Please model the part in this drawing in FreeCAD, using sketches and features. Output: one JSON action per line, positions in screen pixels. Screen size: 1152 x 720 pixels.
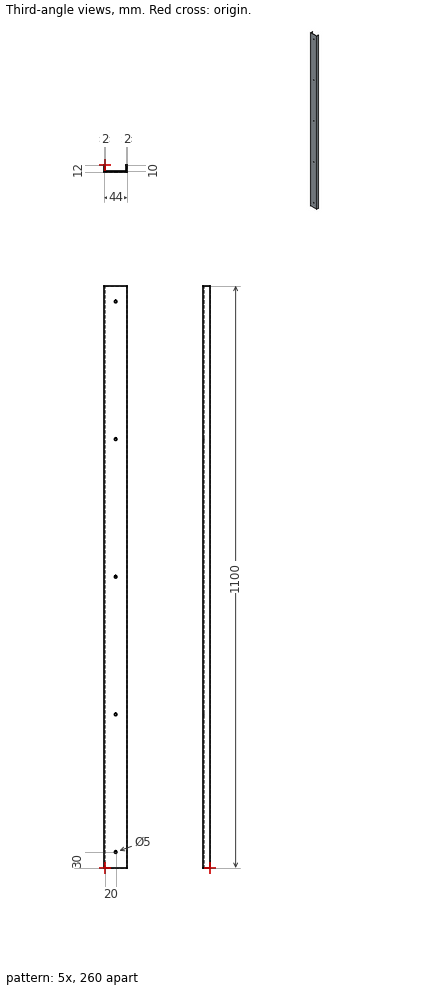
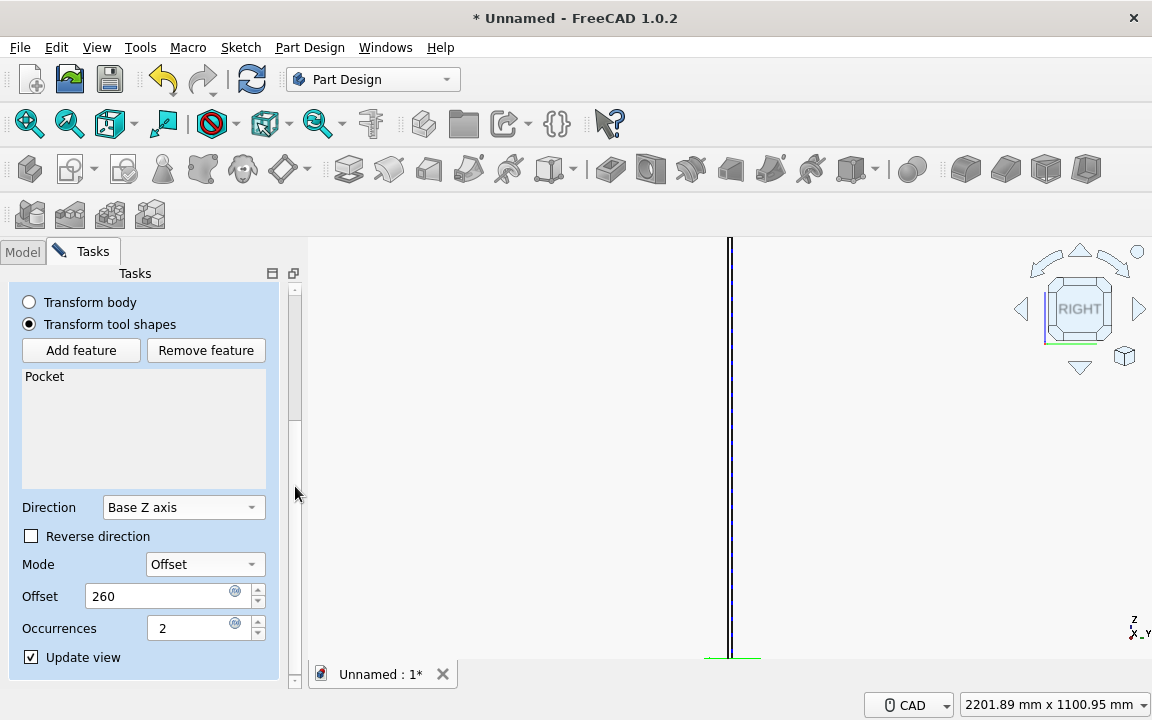
{"action": "triple_click", "coordinate": [198, 628]}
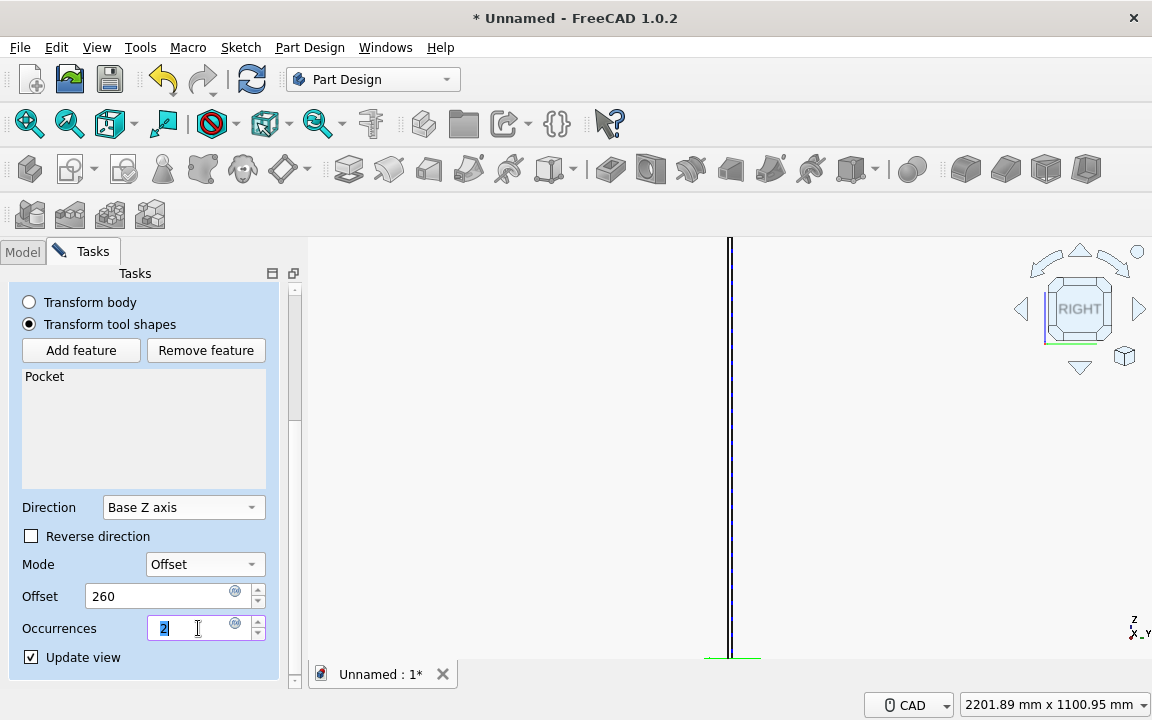
{"action": "type", "text": "5"}
{"action": "key", "text": "Tab"}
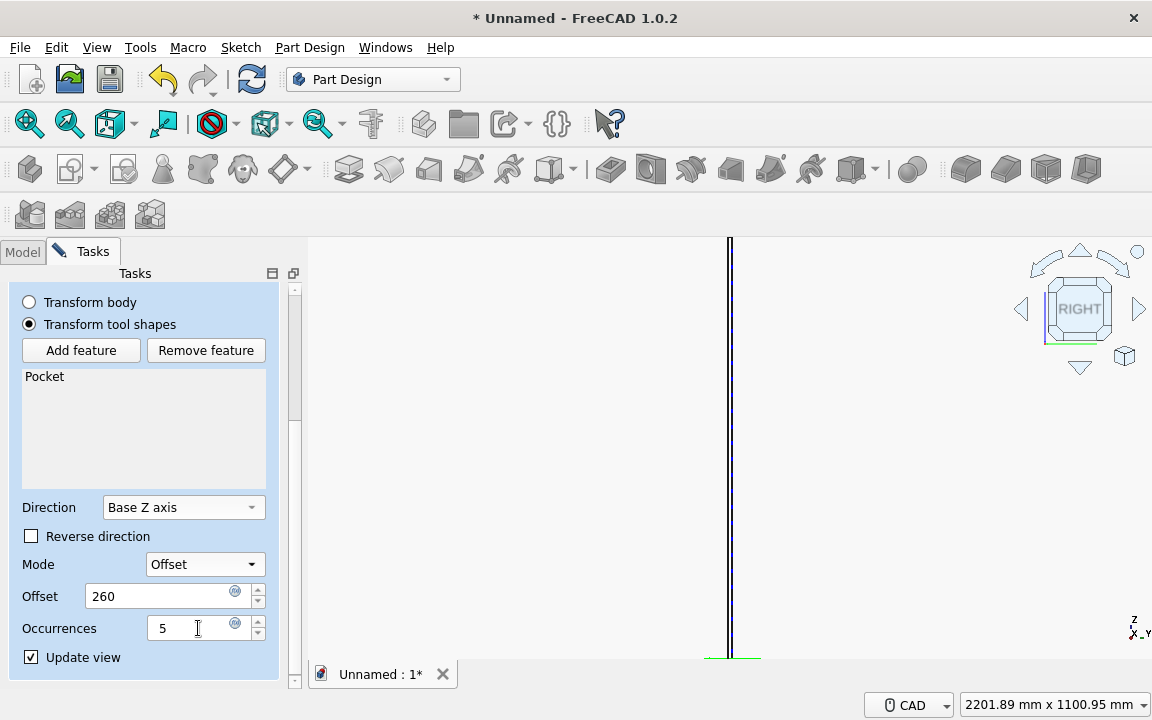
{"action": "scroll", "coordinate": [295, 486], "scroll_direction": "up", "scroll_amount": 5}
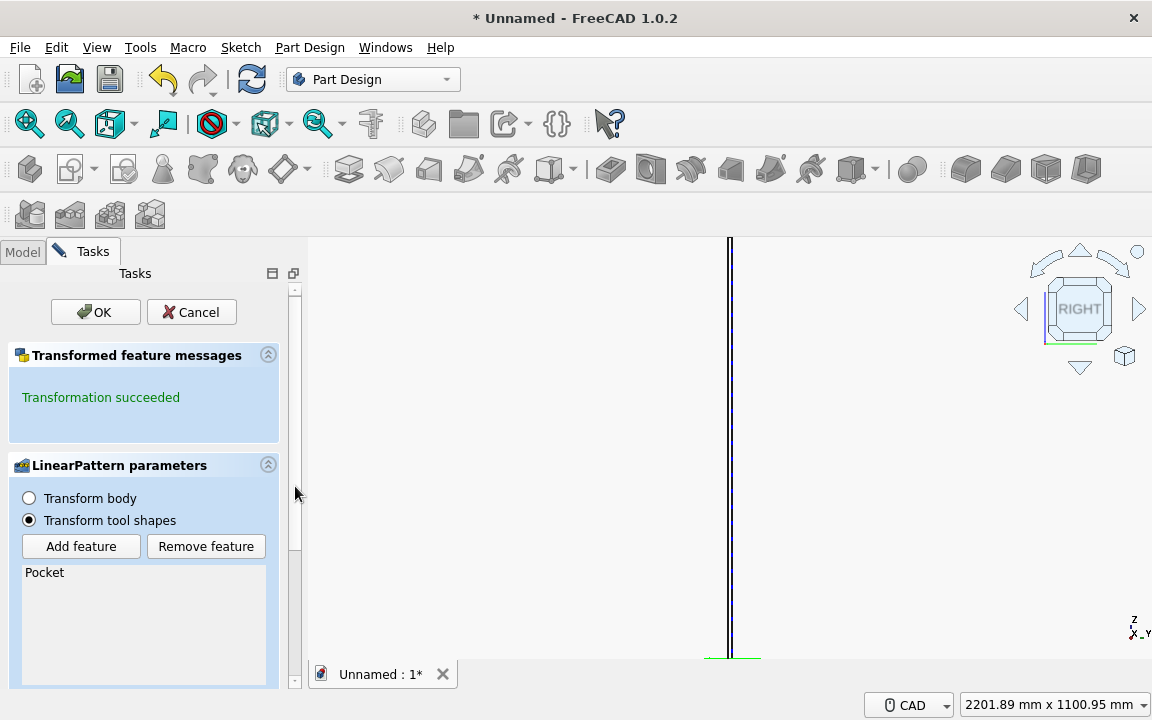
{"action": "left_click", "coordinate": [96, 312]}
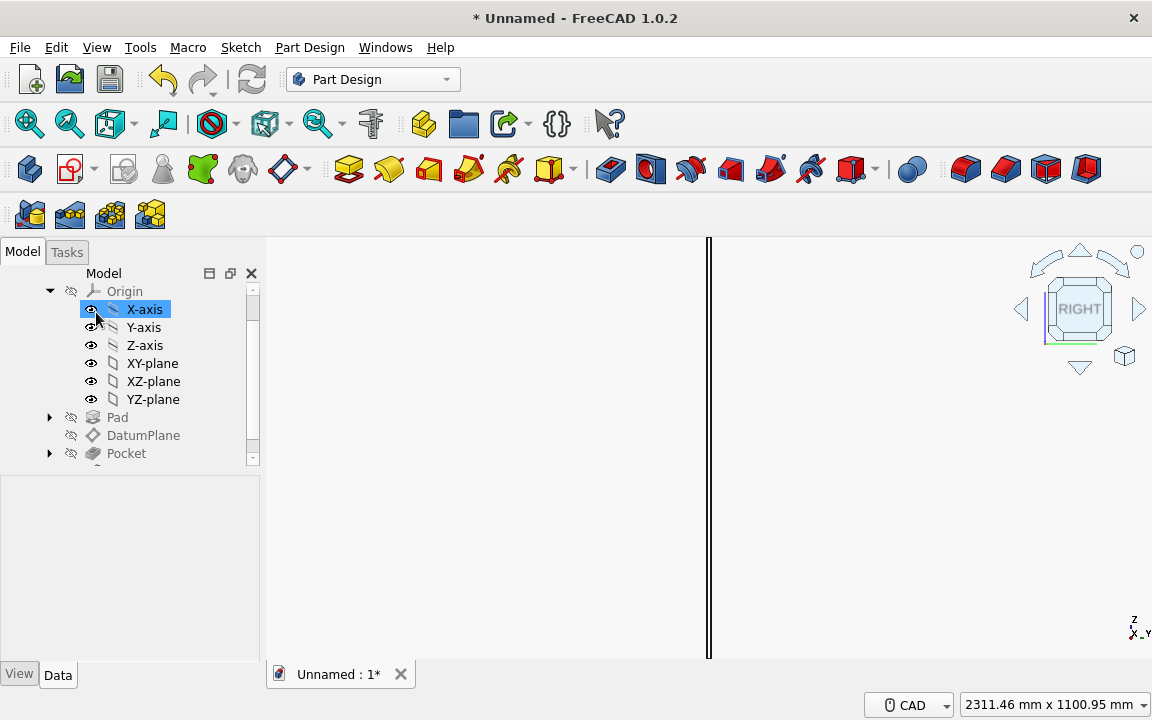
{"action": "key", "text": "0"}